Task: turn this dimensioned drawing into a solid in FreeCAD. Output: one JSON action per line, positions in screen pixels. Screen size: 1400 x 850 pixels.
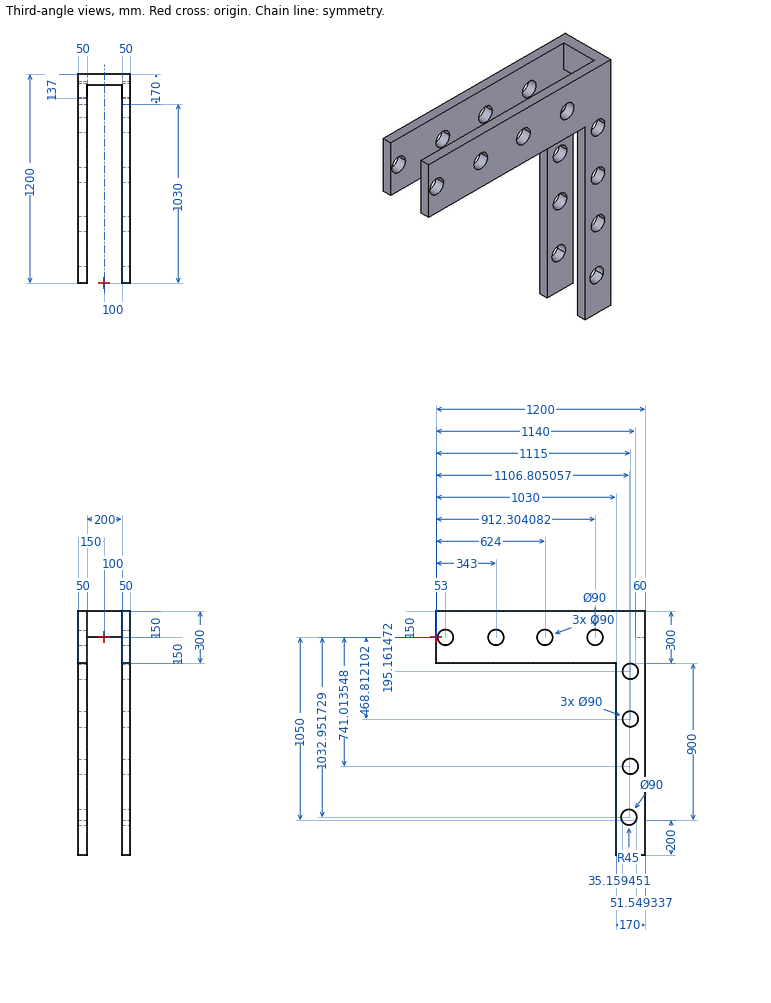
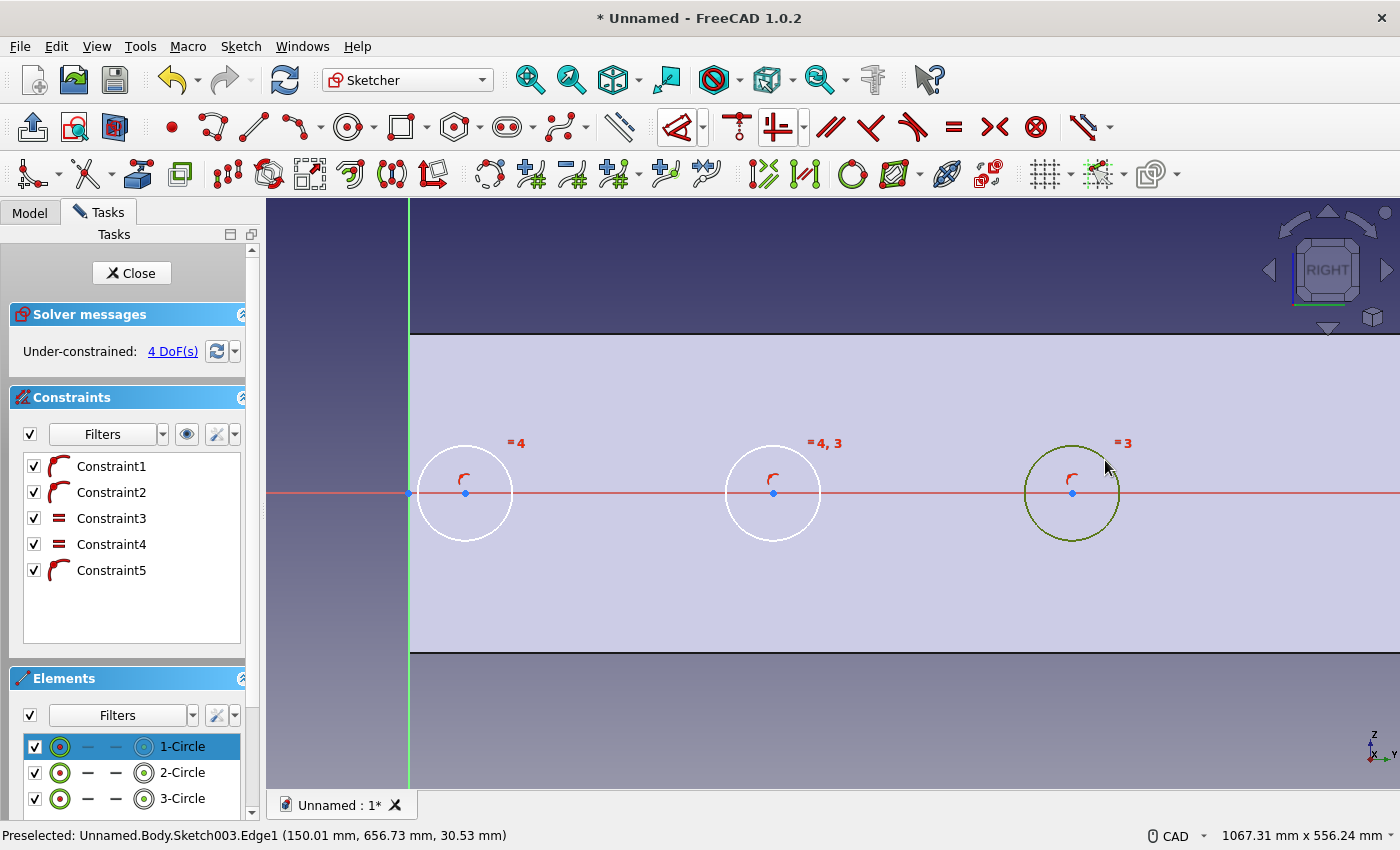
{"action": "left_click", "coordinate": [702, 128]}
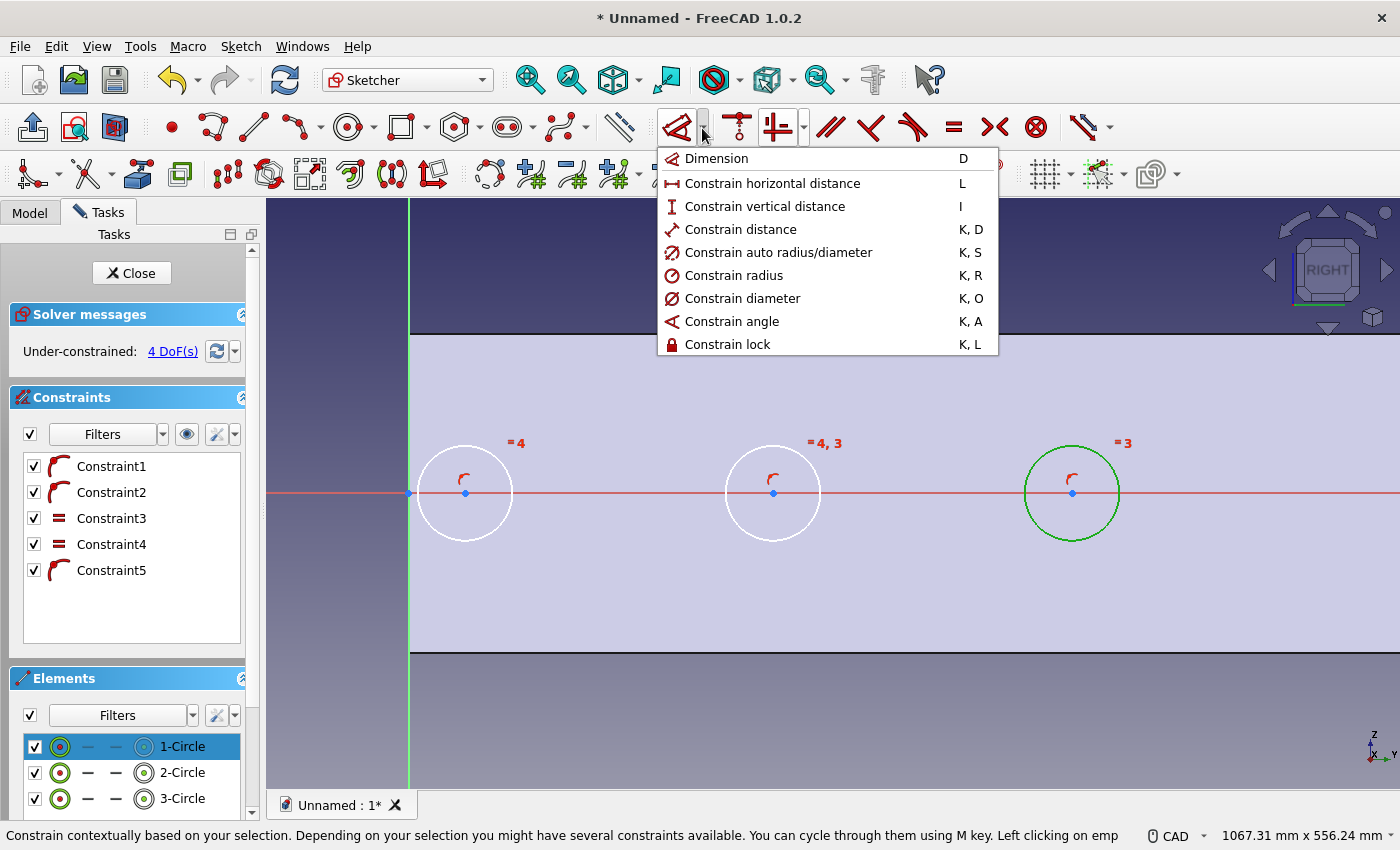
{"action": "left_click", "coordinate": [828, 298]}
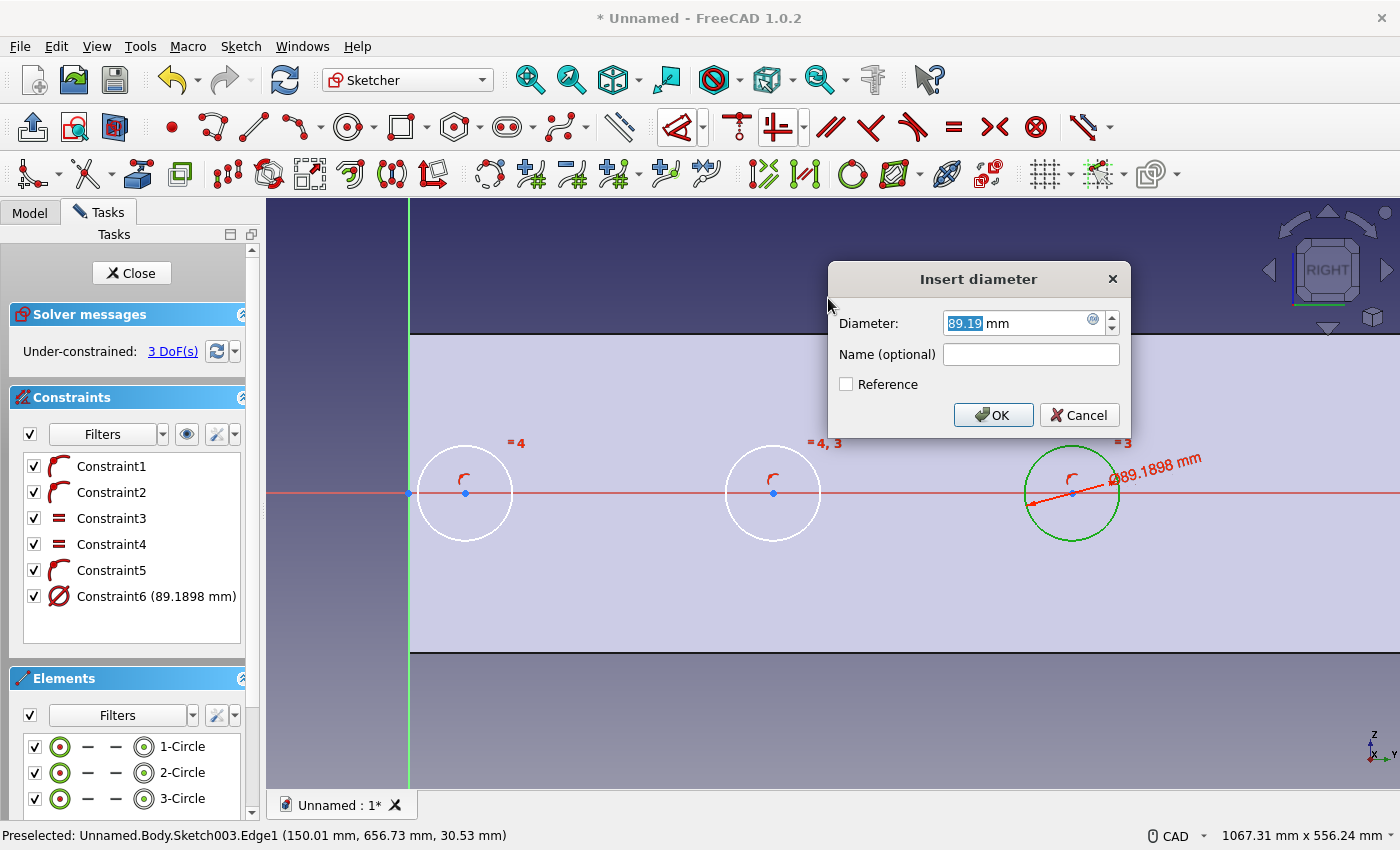
{"action": "type", "text": "90"}
{"action": "key", "text": "Return"}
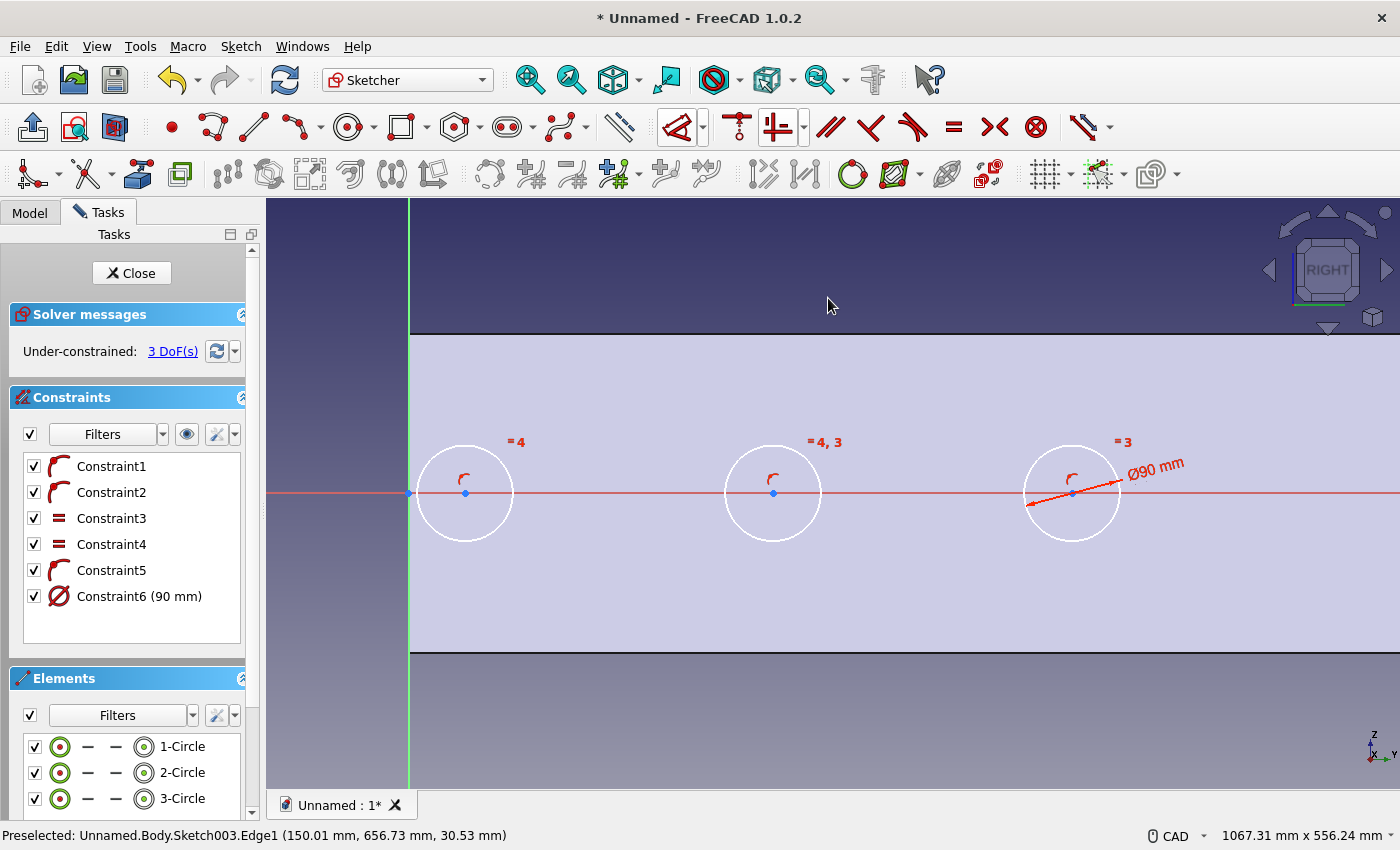
{"action": "left_click", "coordinate": [465, 493]}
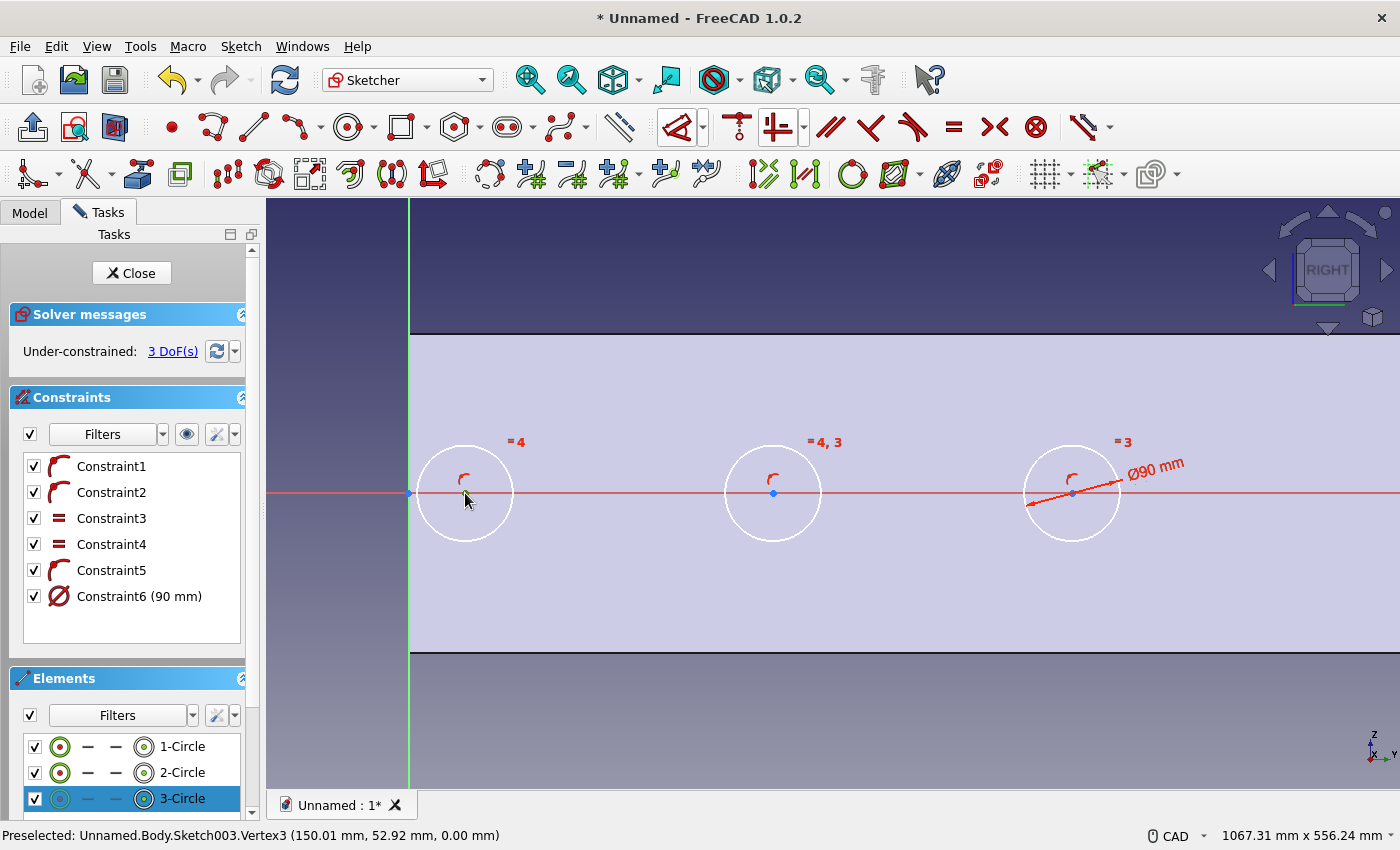
{"action": "key", "text": "l"}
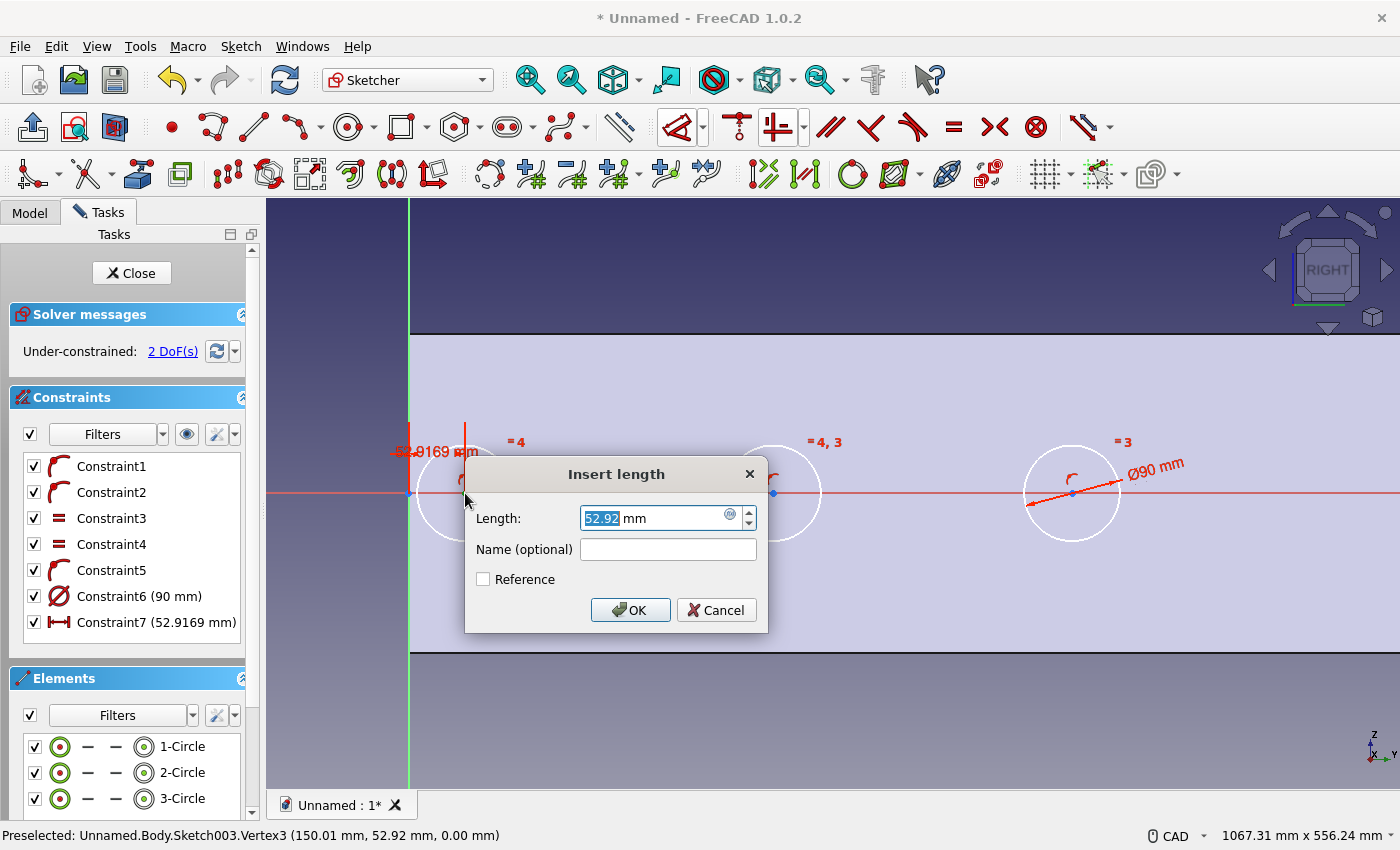
{"action": "type", "text": "53"}
{"action": "key", "text": "Return"}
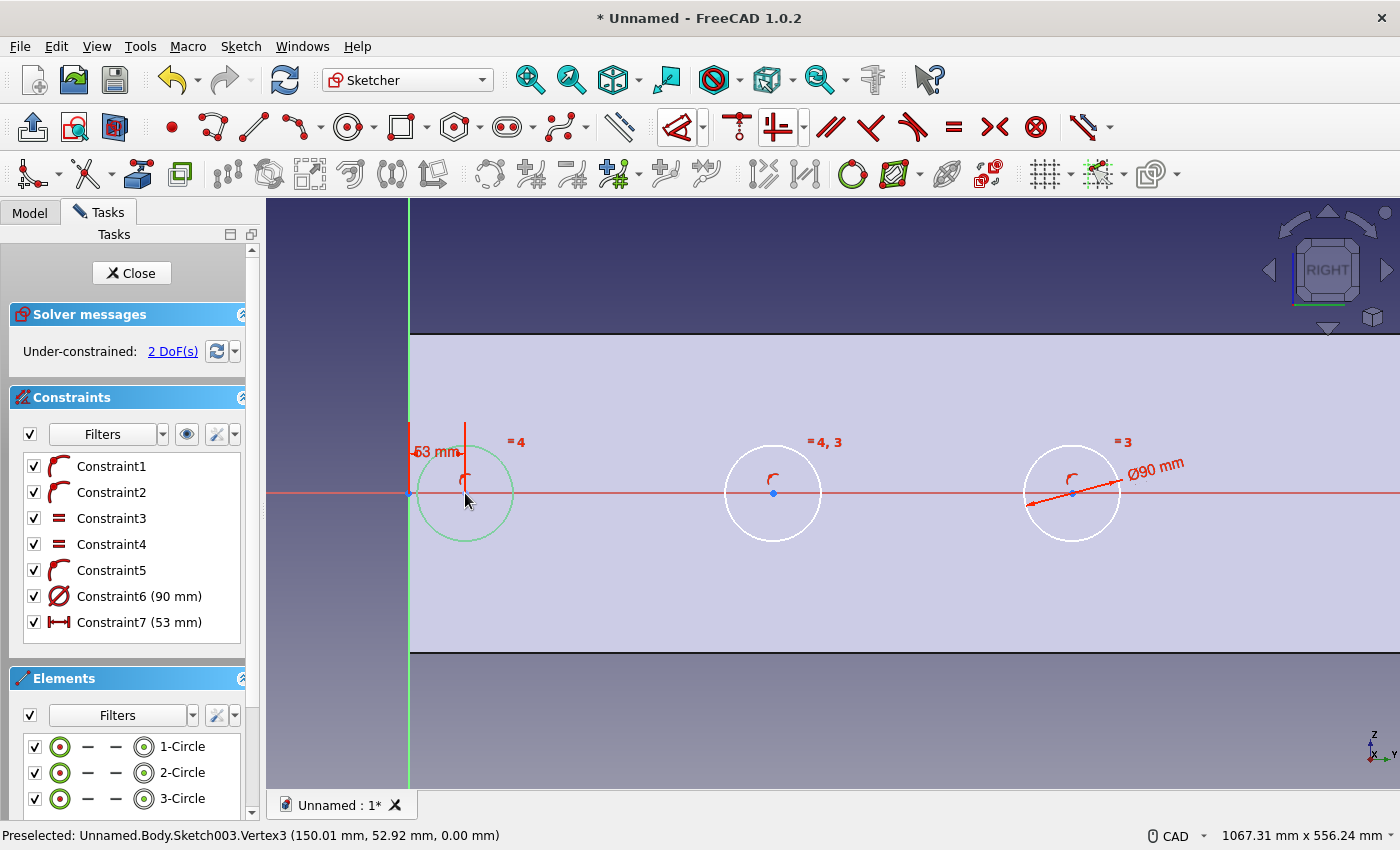
{"action": "left_click", "coordinate": [1072, 493]}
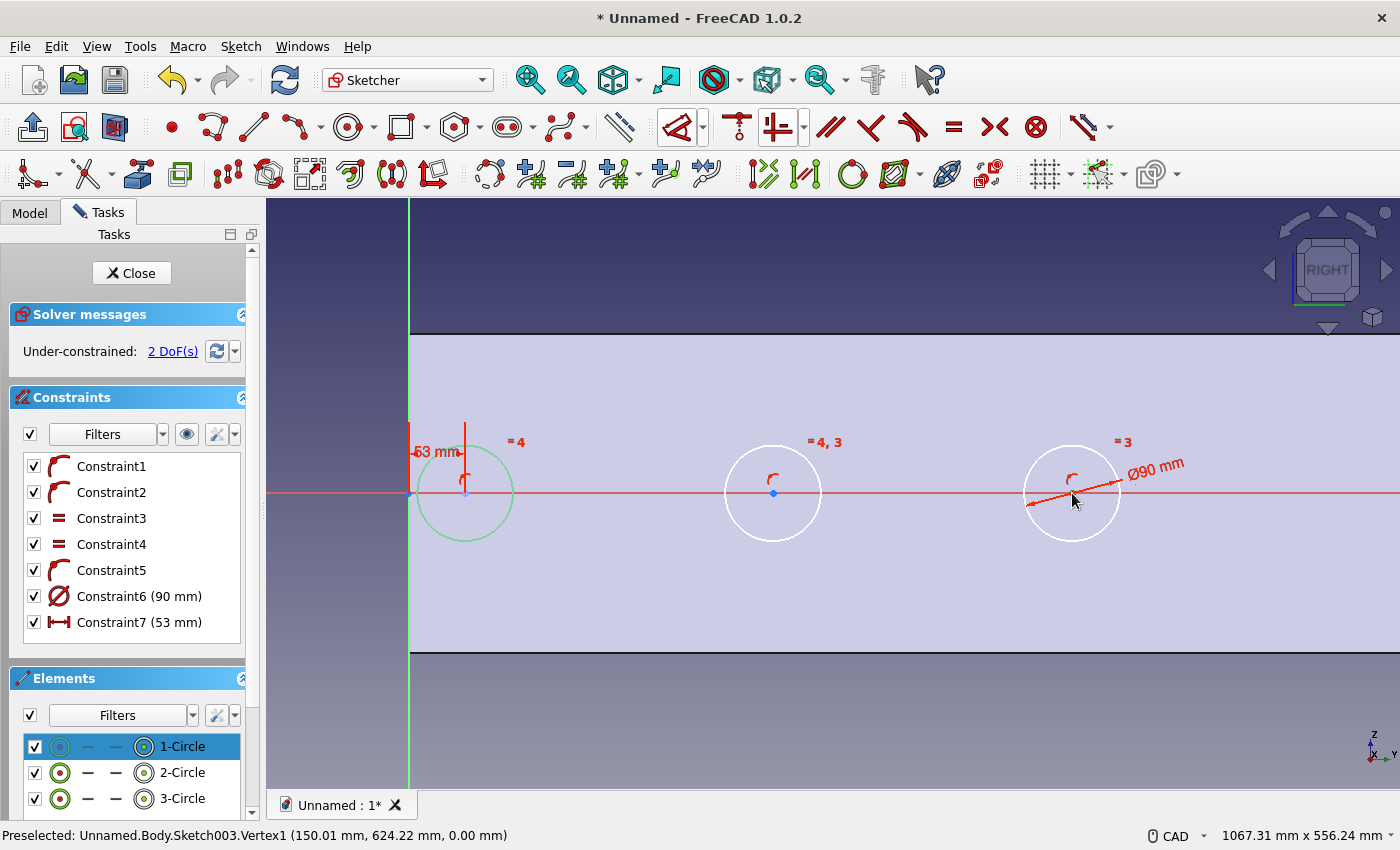
{"action": "left_click", "coordinate": [702, 128]}